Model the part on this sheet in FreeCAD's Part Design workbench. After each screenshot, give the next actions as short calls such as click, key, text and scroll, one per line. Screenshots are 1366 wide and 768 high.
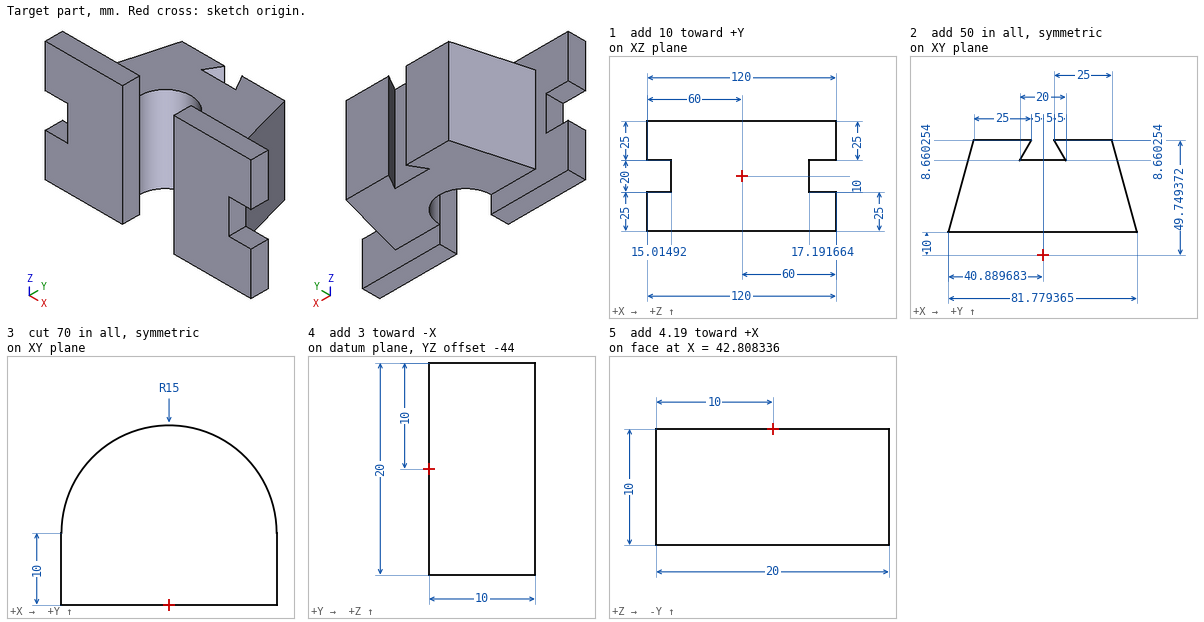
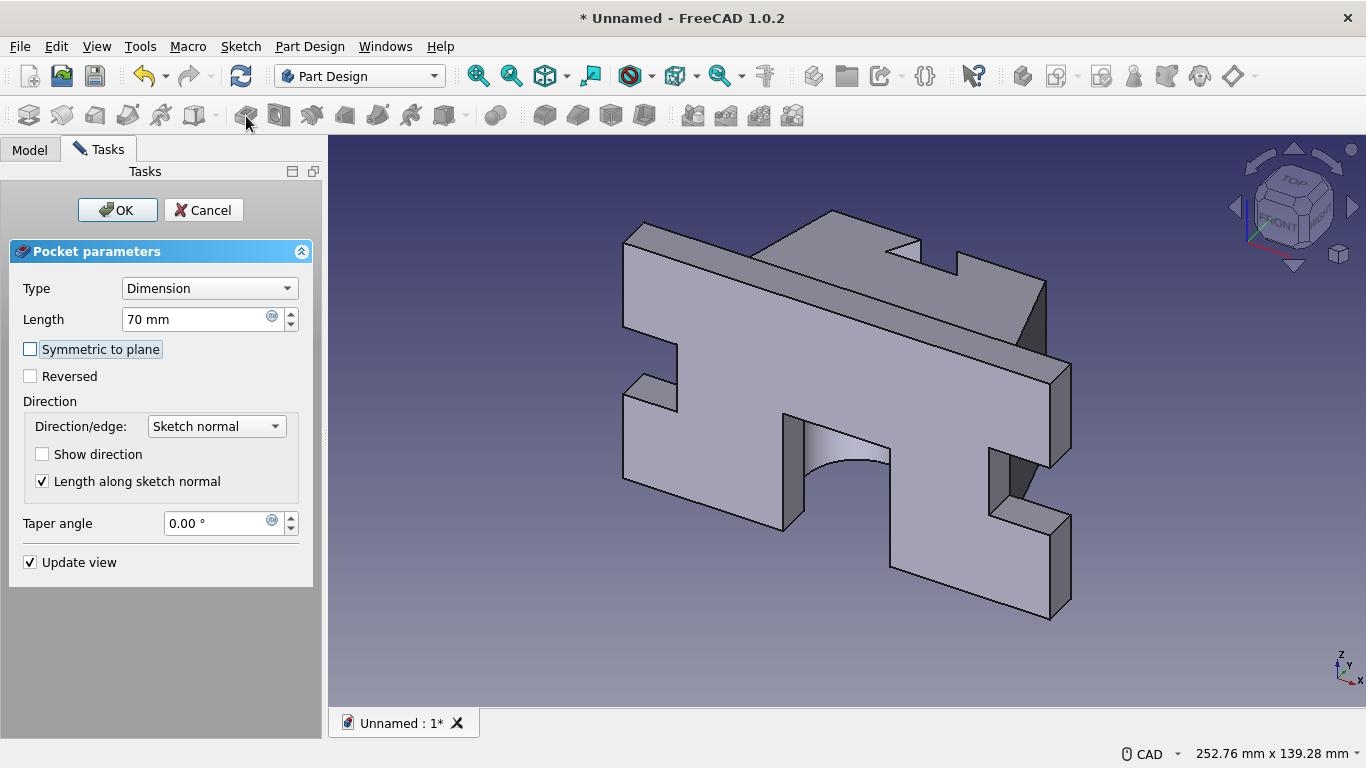
click(31, 349)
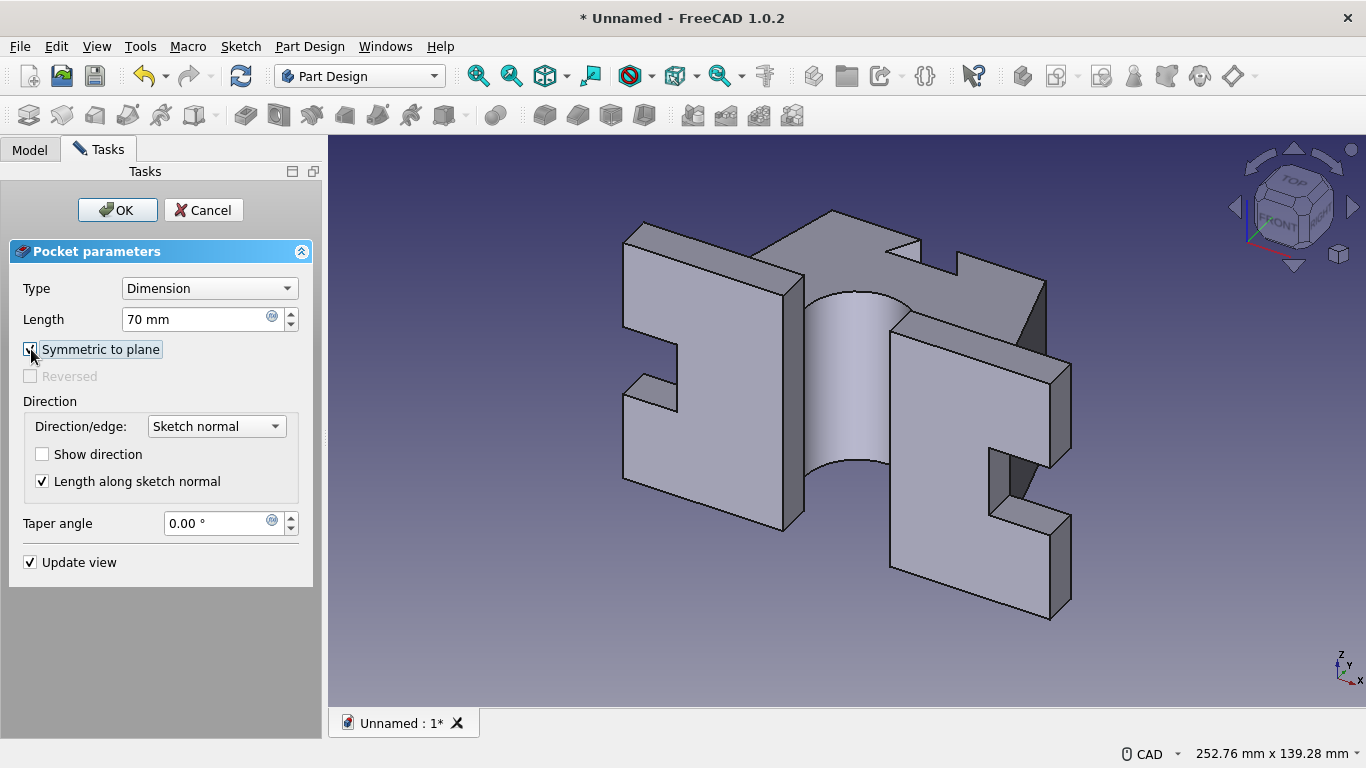
click(118, 210)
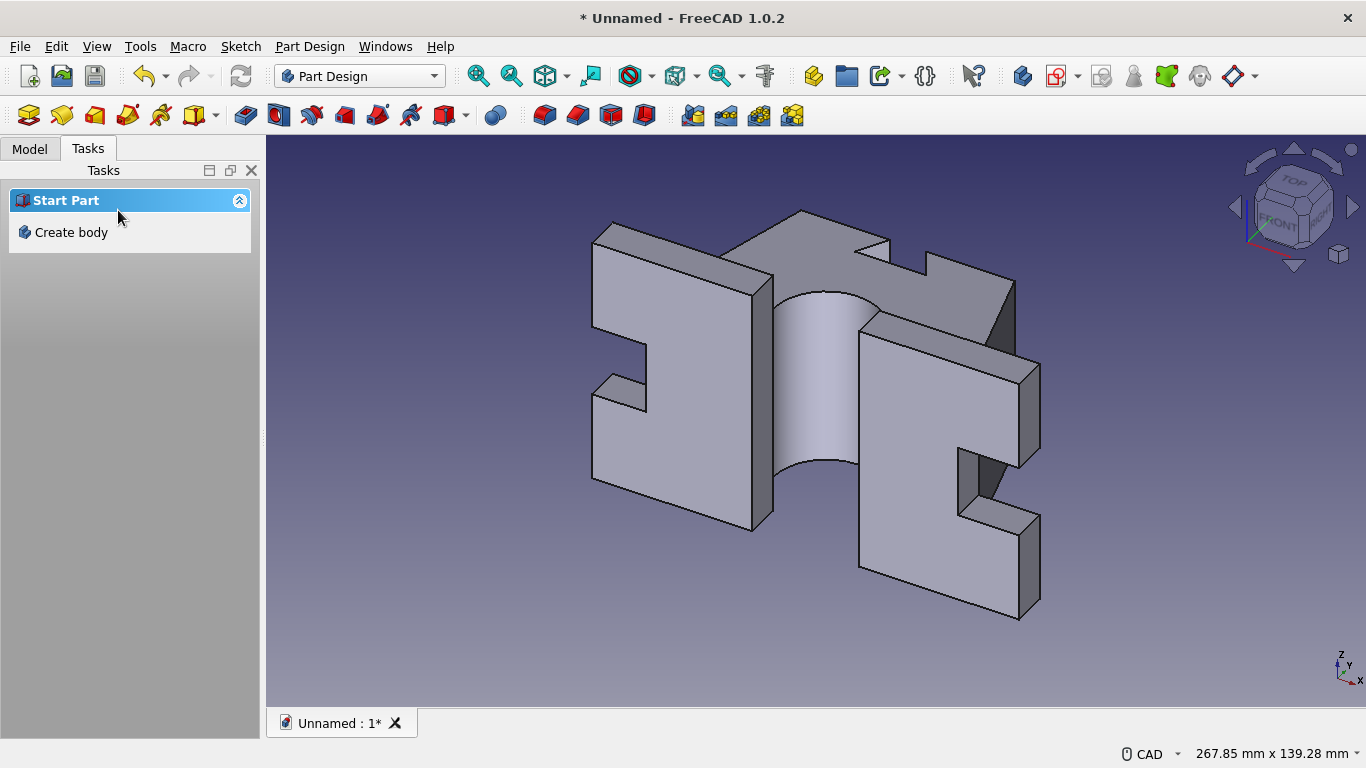
click(30, 148)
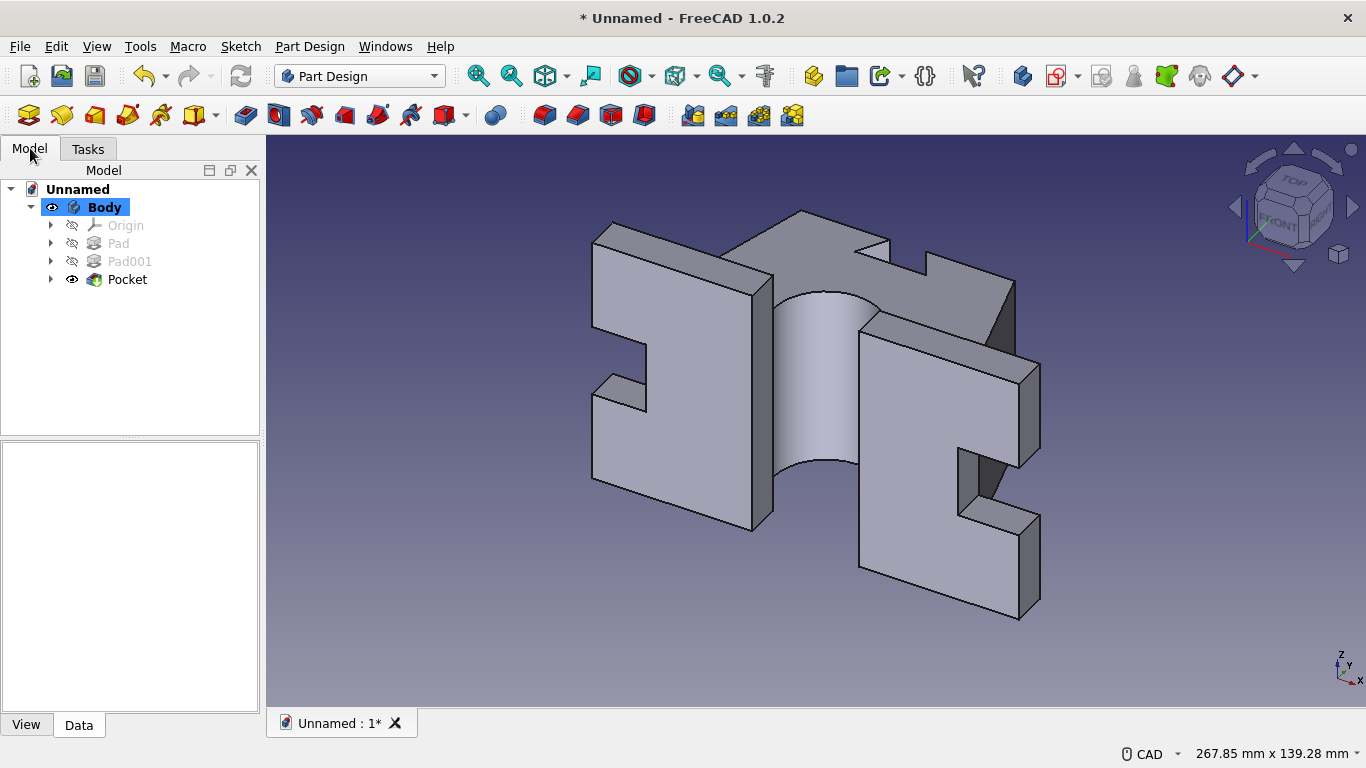
click(51, 225)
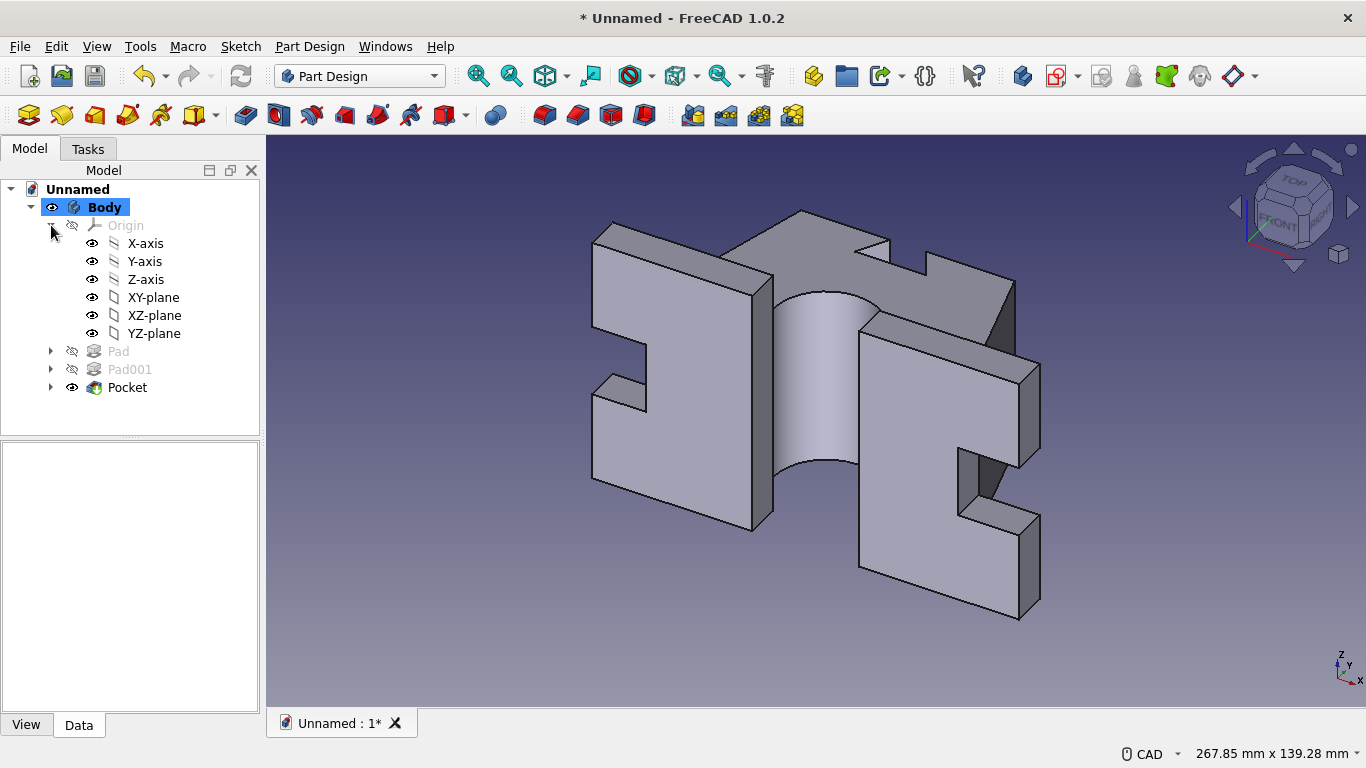
click(137, 333)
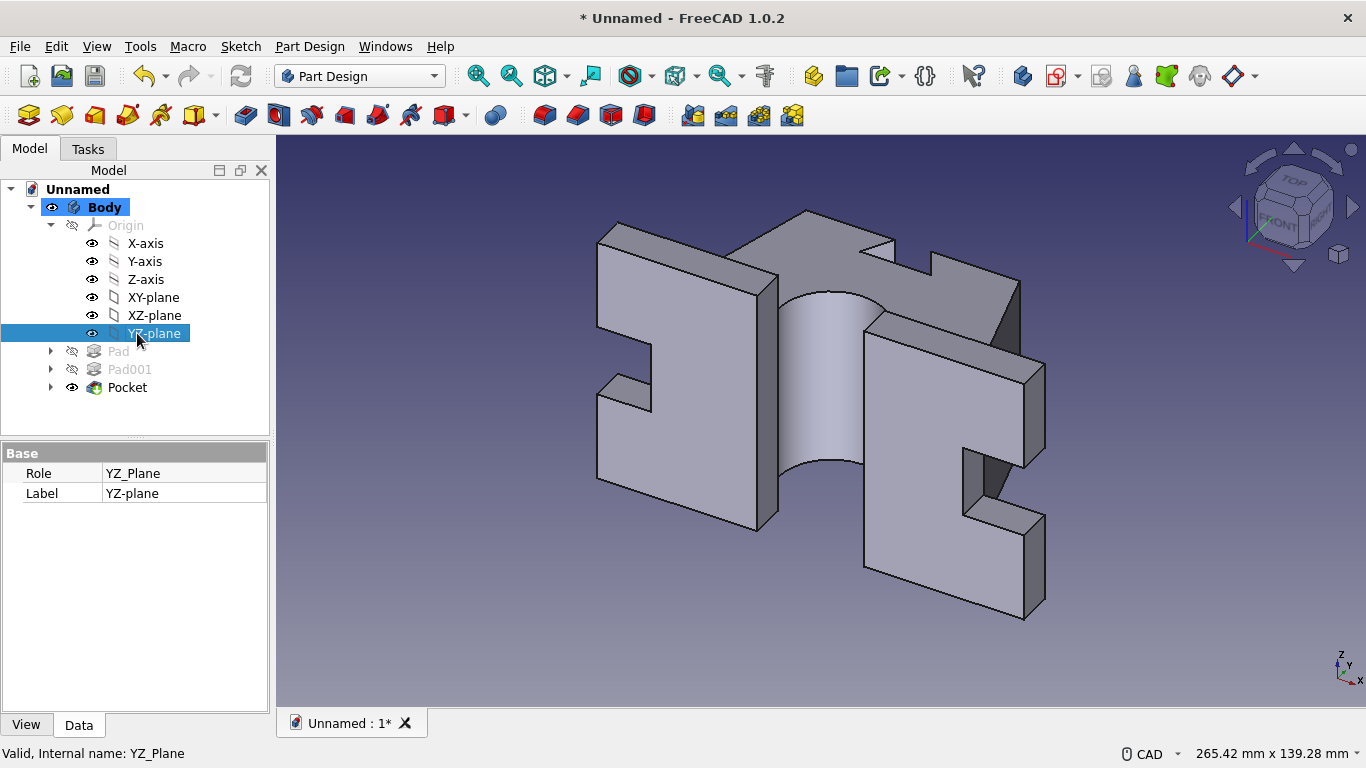
click(1232, 76)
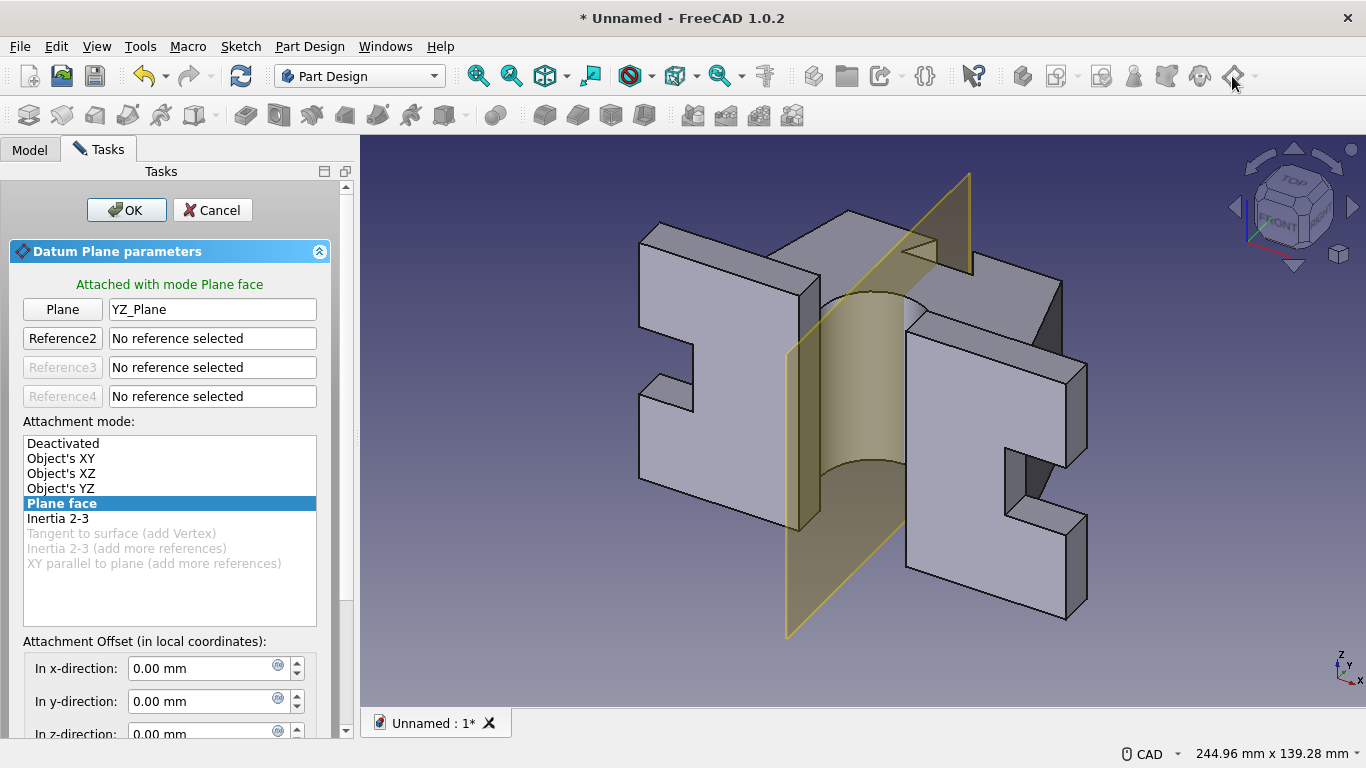
scroll(346, 460, down, 2)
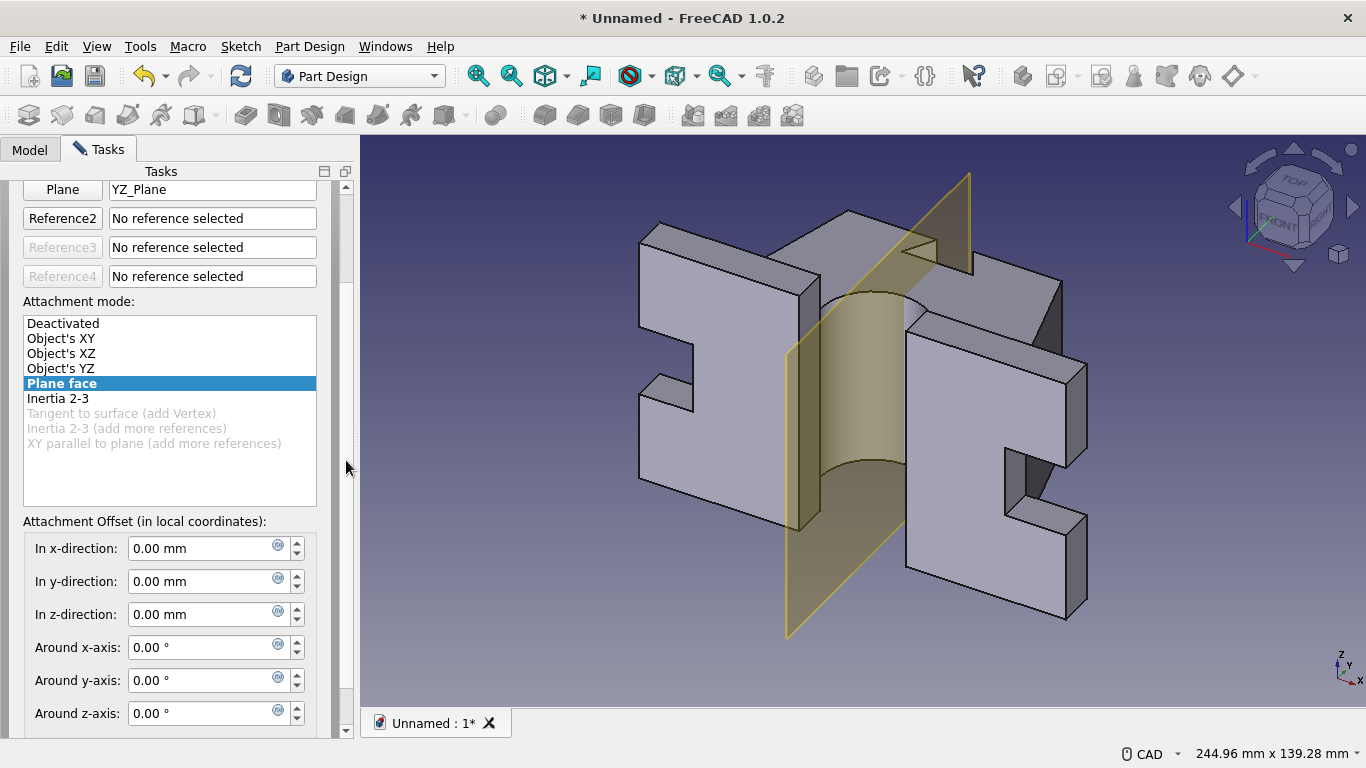
triple_click(210, 614)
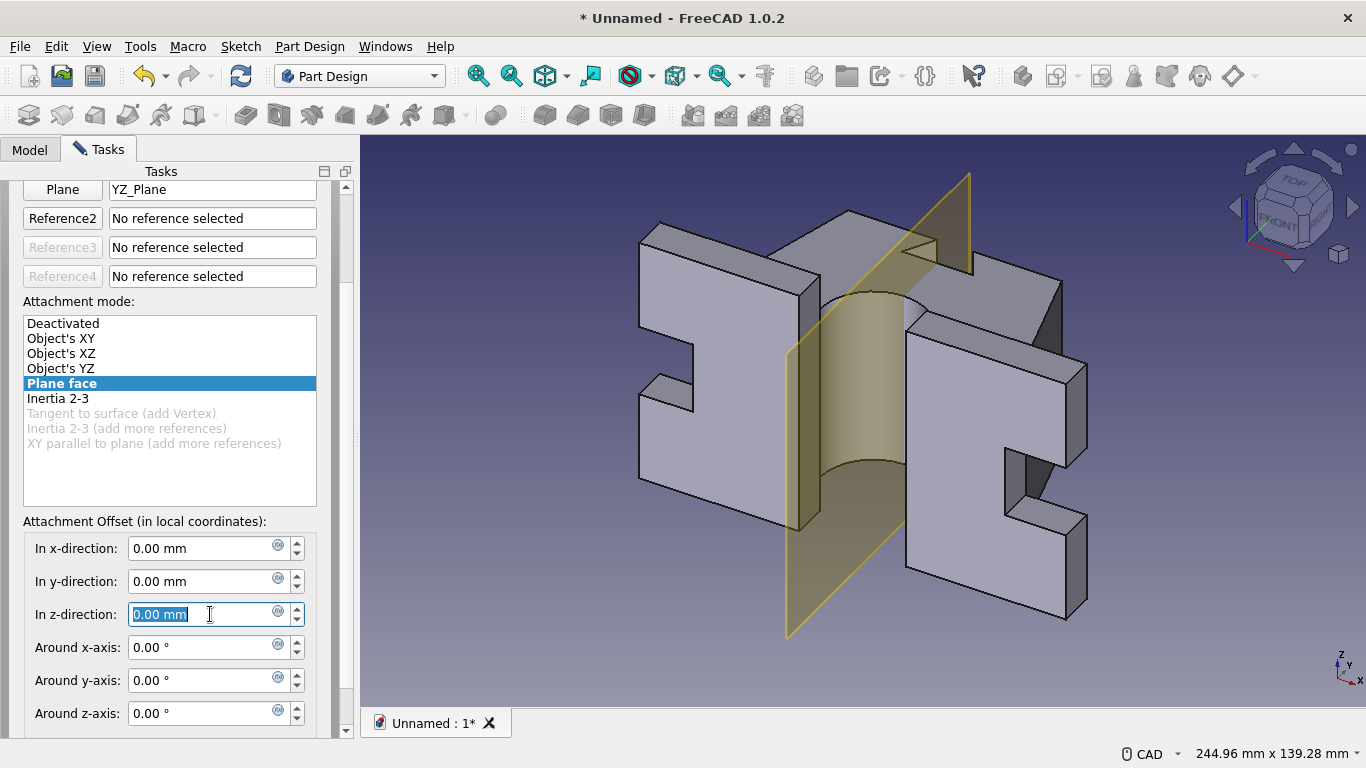
text(-44)
key(Tab)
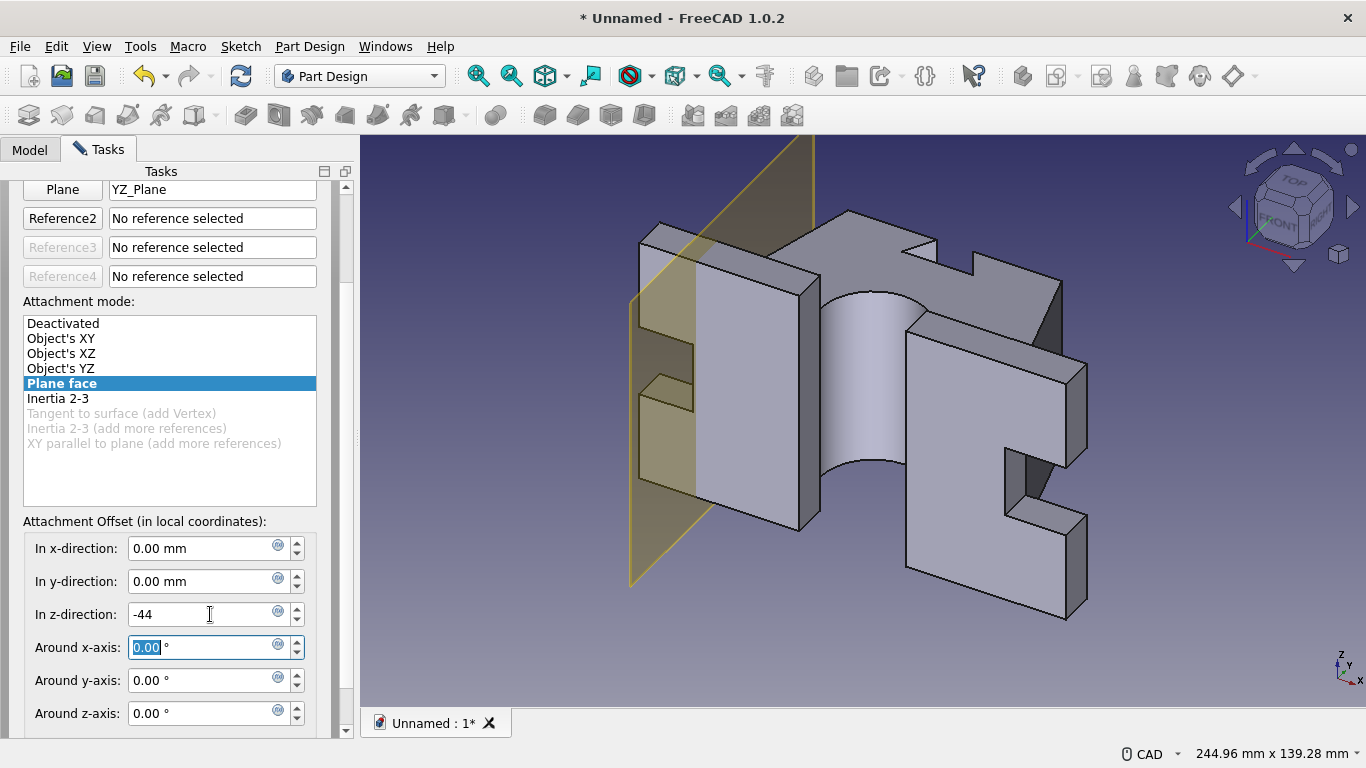
scroll(346, 460, up, 3)